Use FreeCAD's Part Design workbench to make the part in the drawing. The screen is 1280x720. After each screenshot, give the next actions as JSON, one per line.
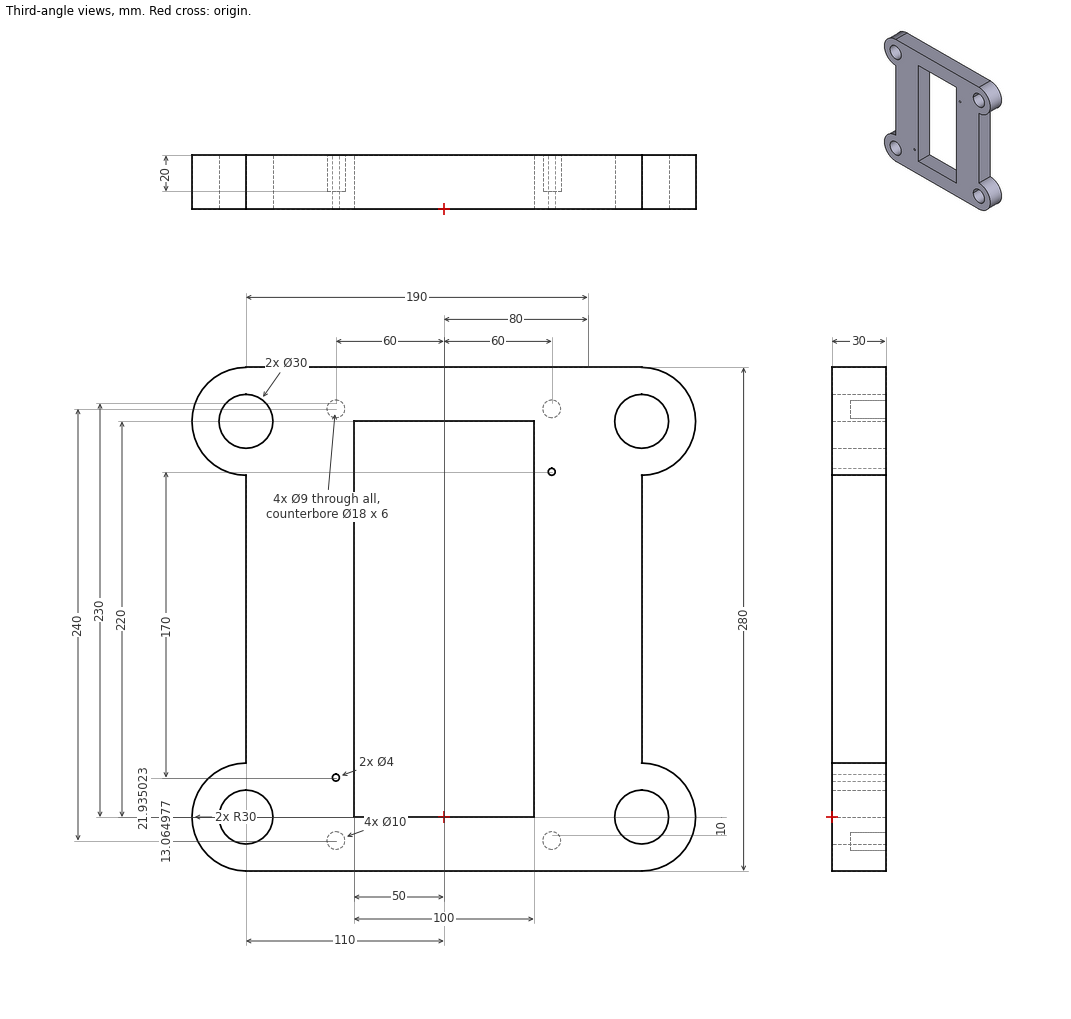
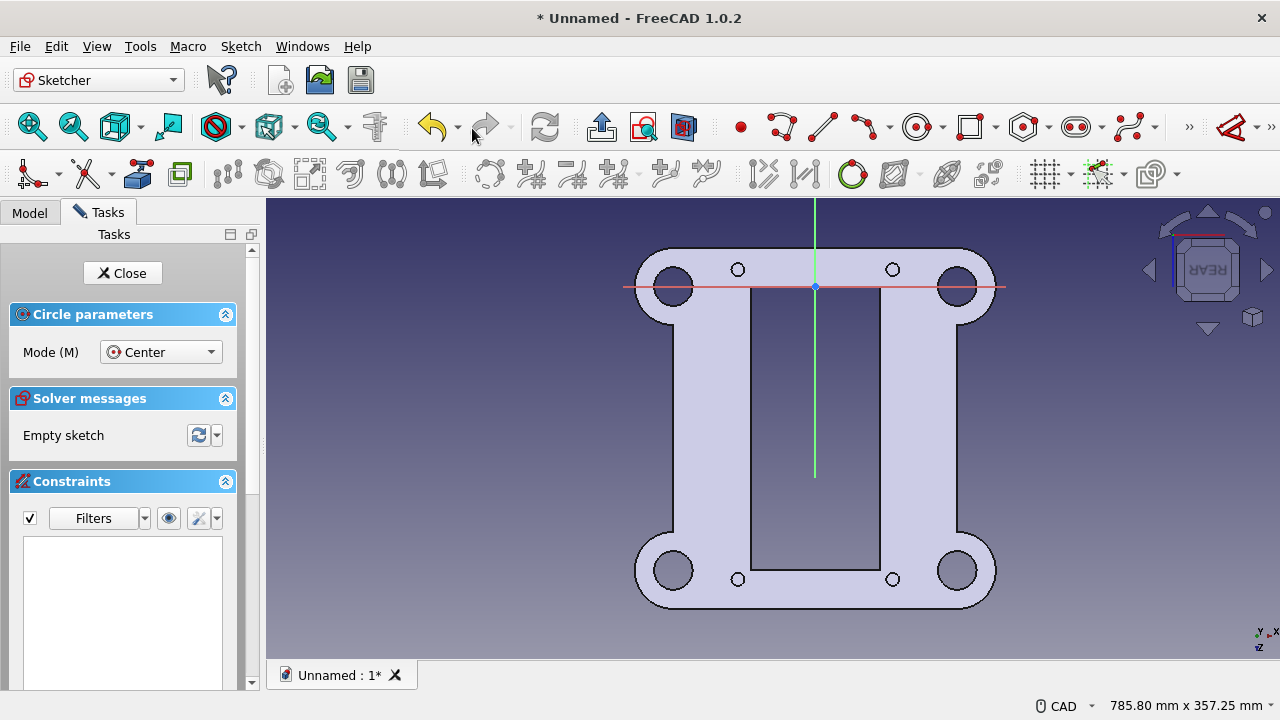
{"action": "scroll", "coordinate": [738, 315], "scroll_direction": "up", "scroll_amount": 11}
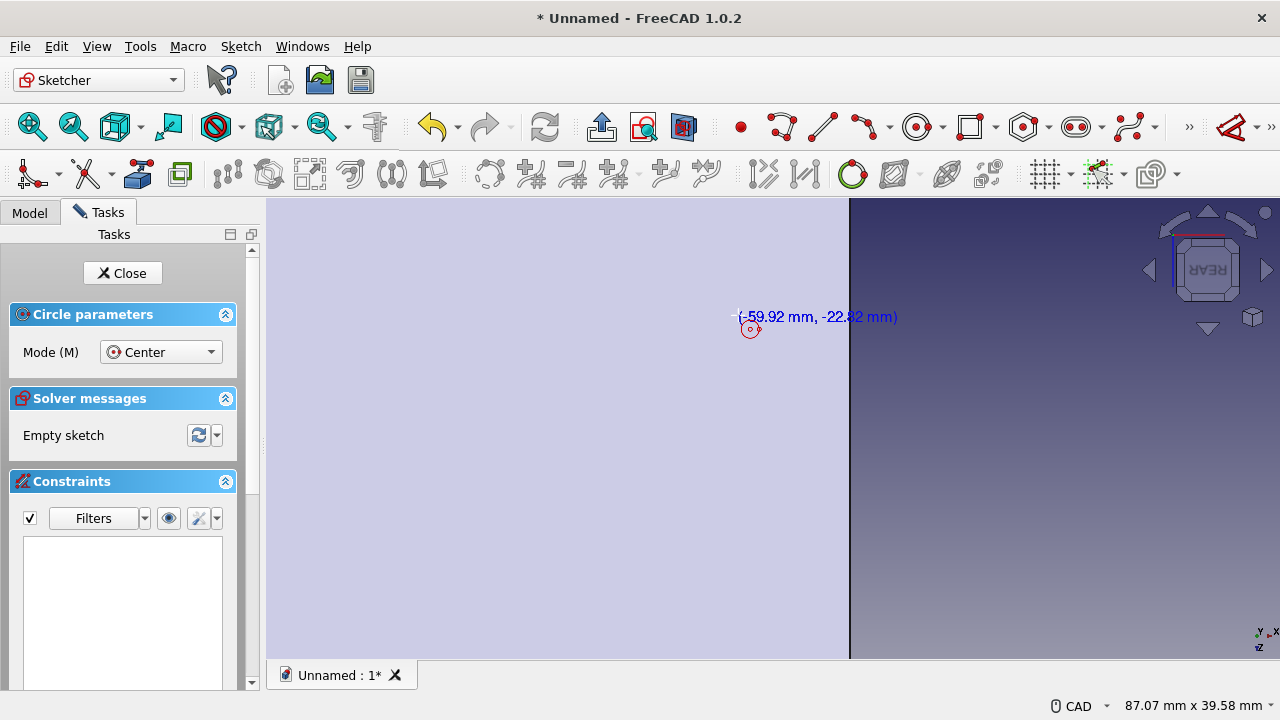
{"action": "scroll", "coordinate": [591, 310], "scroll_direction": "down", "scroll_amount": 10}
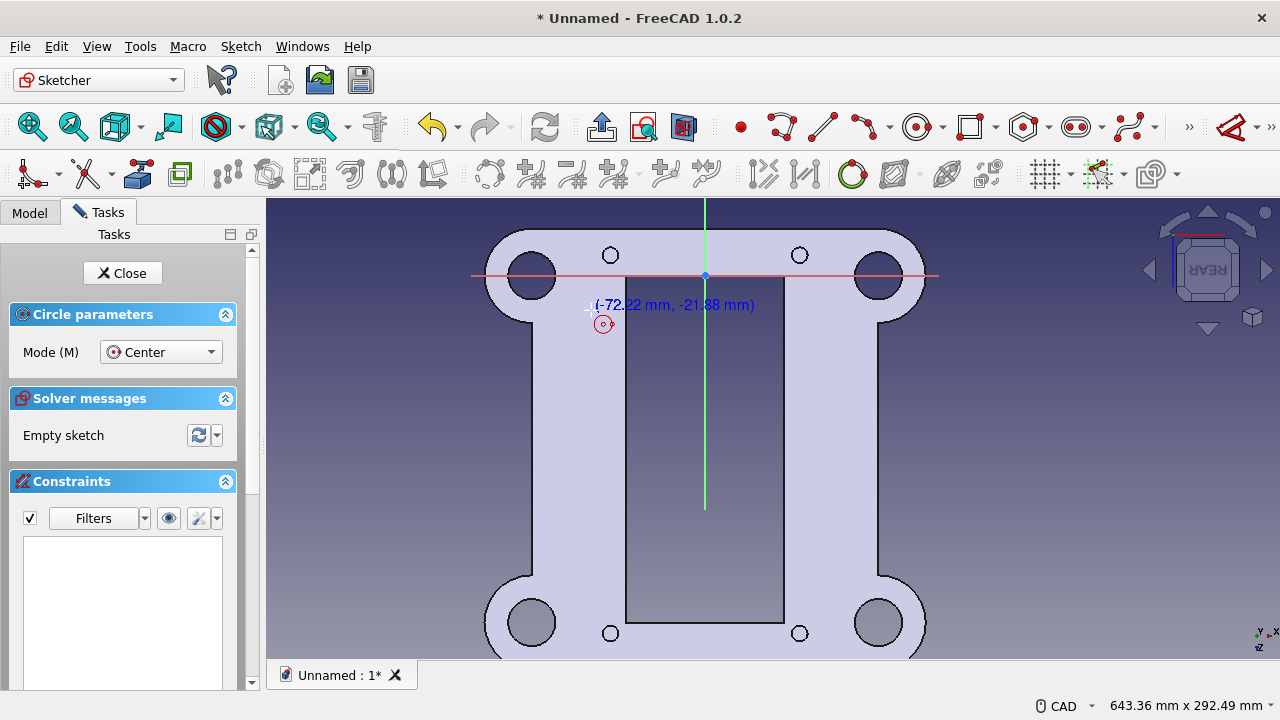
{"action": "left_click", "coordinate": [611, 310]}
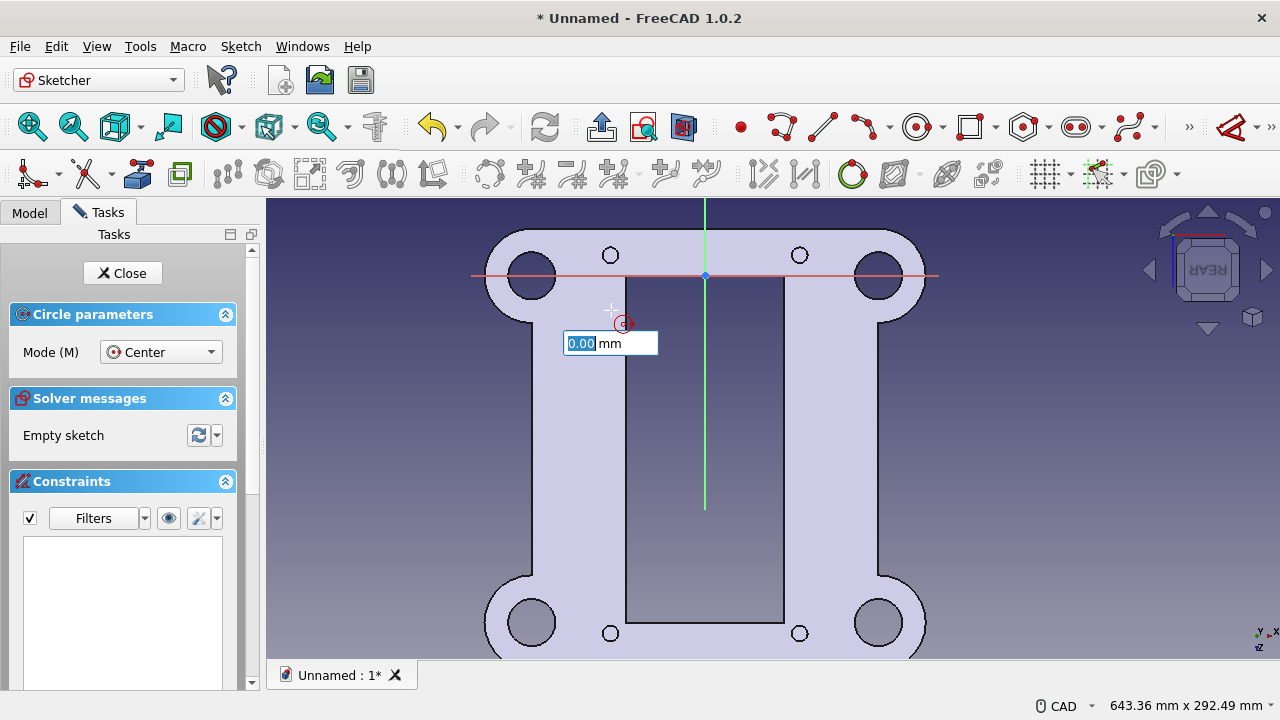
{"action": "scroll", "coordinate": [613, 308], "scroll_direction": "up", "scroll_amount": 9}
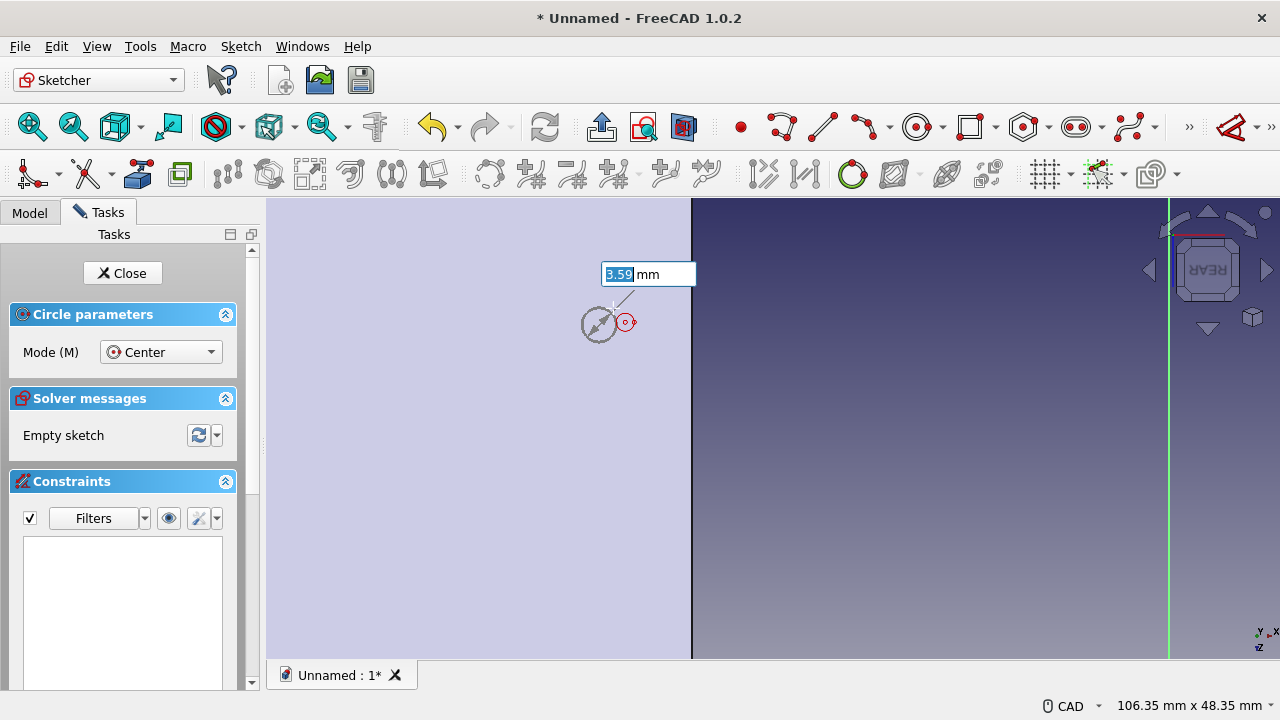
{"action": "left_click", "coordinate": [610, 308]}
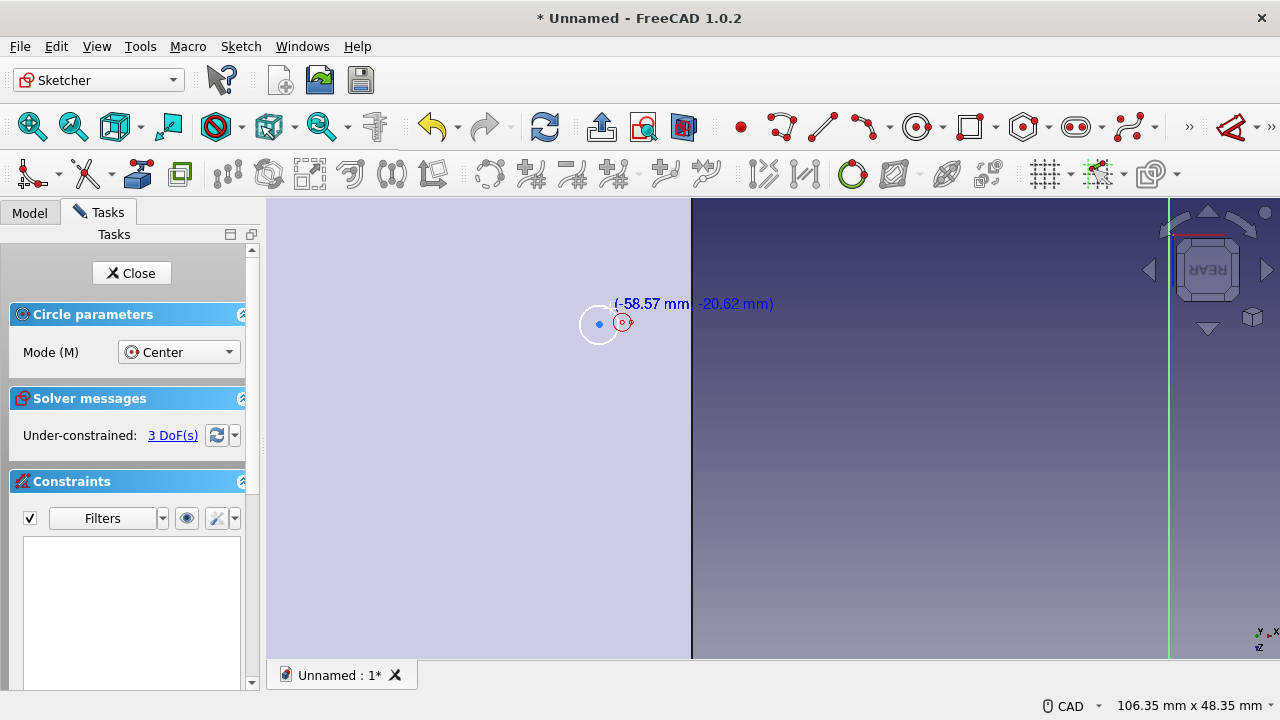
{"action": "scroll", "coordinate": [613, 308], "scroll_direction": "down", "scroll_amount": 9}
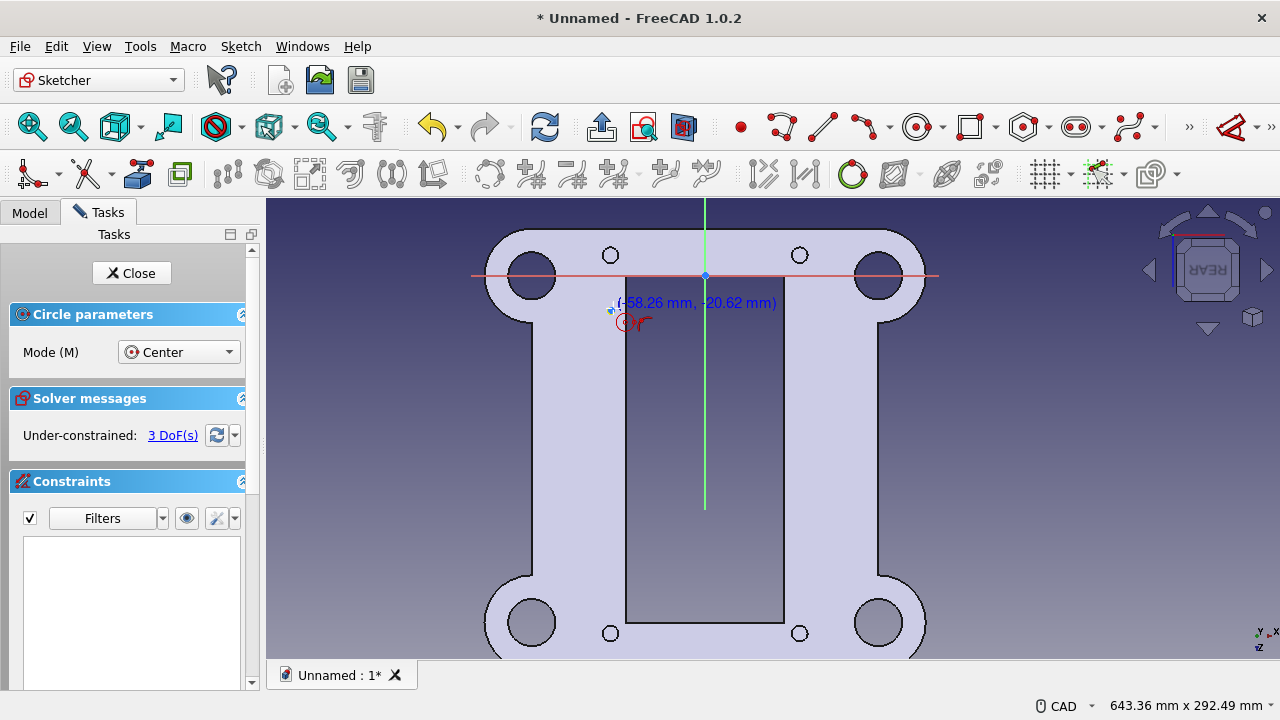
{"action": "scroll", "coordinate": [800, 578], "scroll_direction": "up", "scroll_amount": 10}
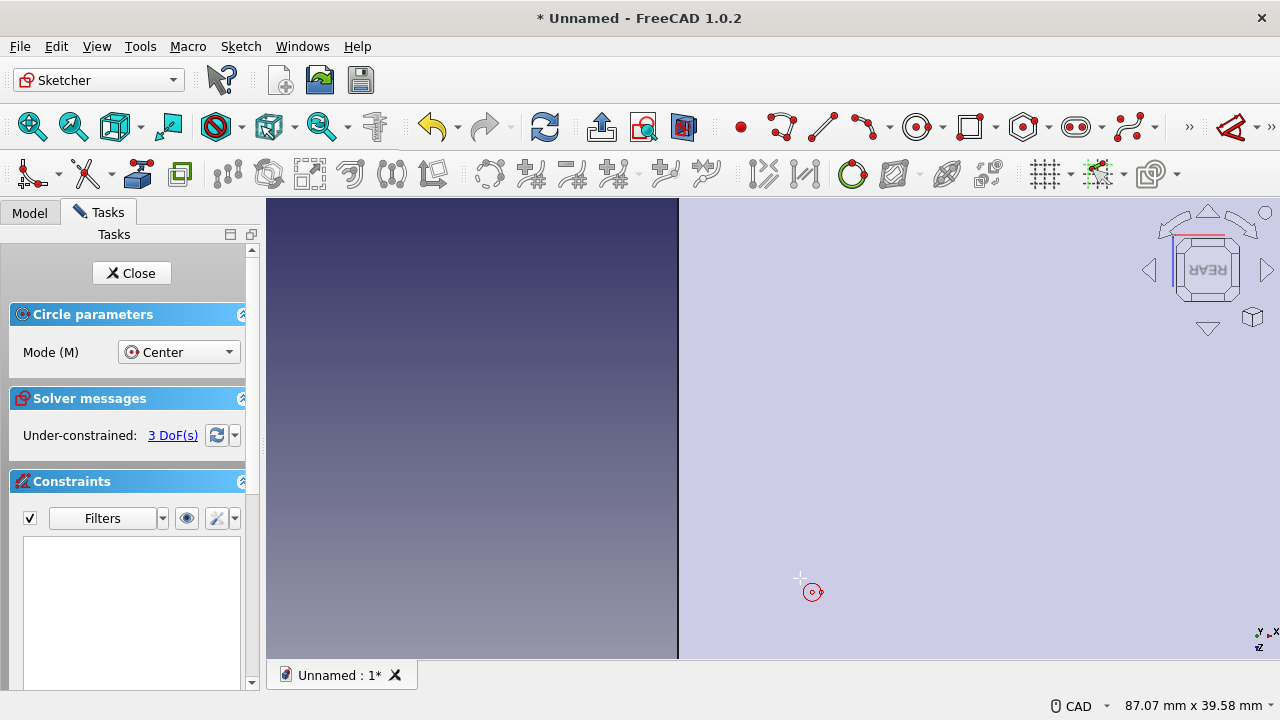
{"action": "scroll", "coordinate": [800, 579], "scroll_direction": "down", "scroll_amount": 10}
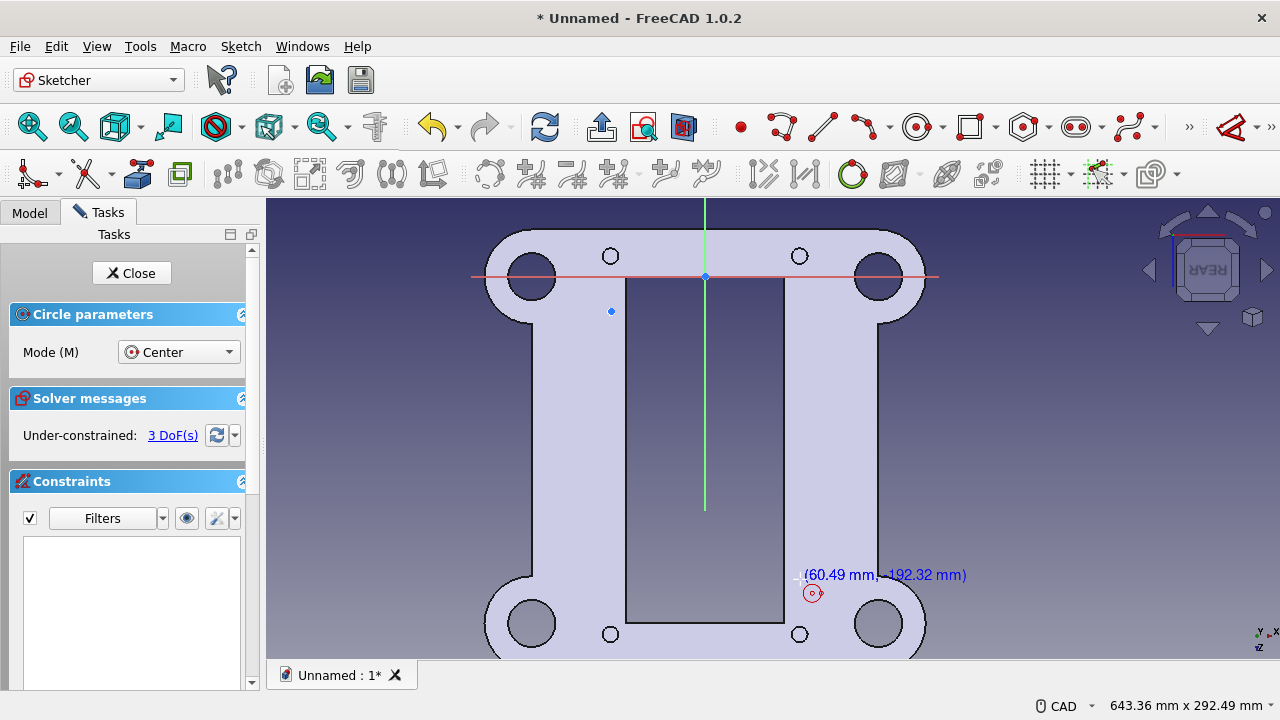
{"action": "left_click", "coordinate": [800, 579]}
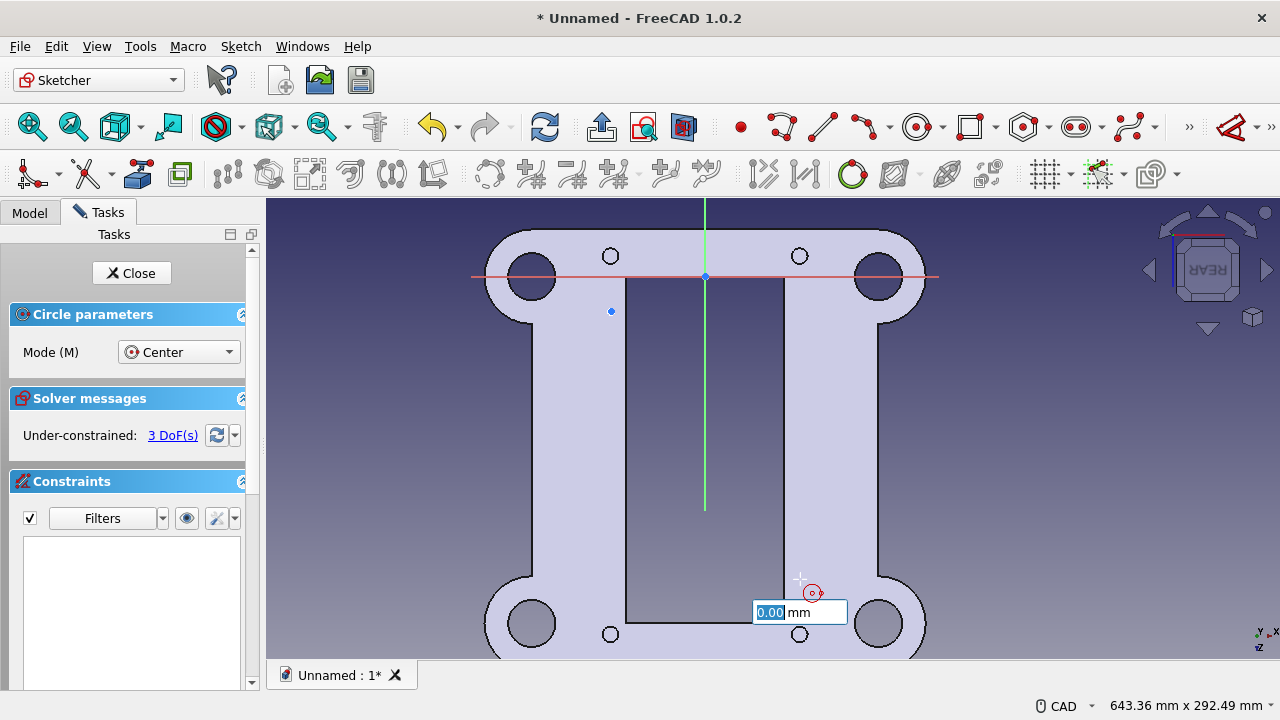
{"action": "scroll", "coordinate": [802, 577], "scroll_direction": "up", "scroll_amount": 9}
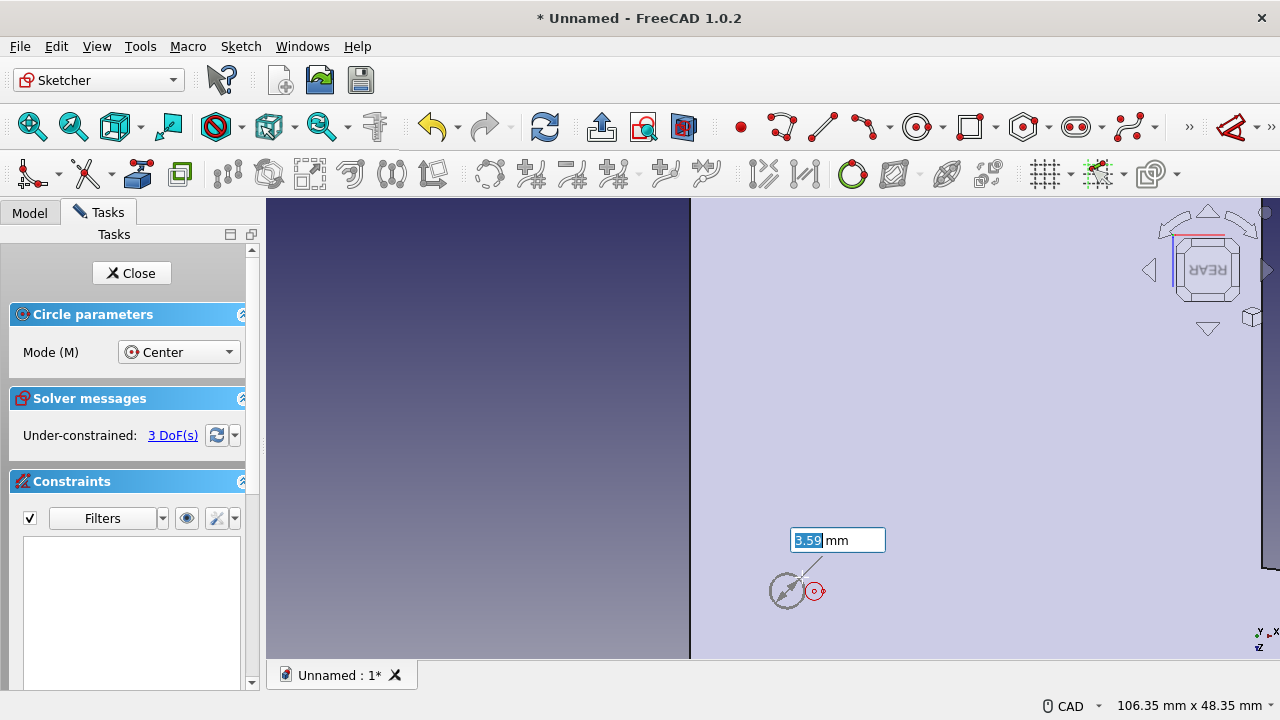
{"action": "left_click", "coordinate": [799, 573]}
{"action": "key", "text": "Escape"}